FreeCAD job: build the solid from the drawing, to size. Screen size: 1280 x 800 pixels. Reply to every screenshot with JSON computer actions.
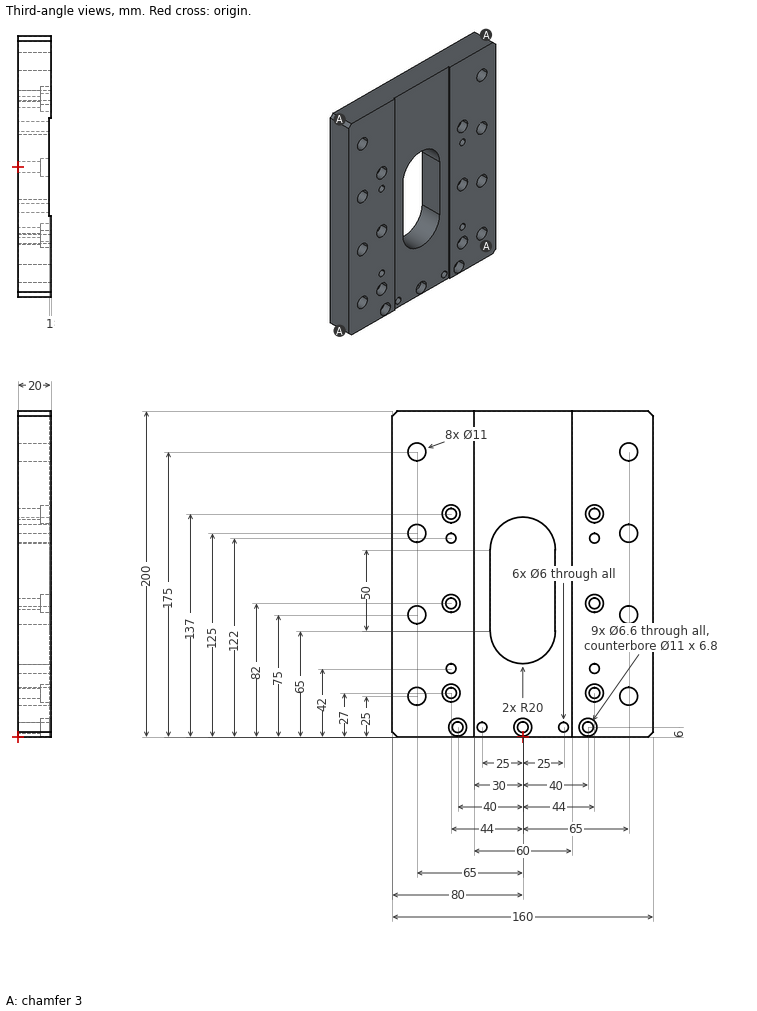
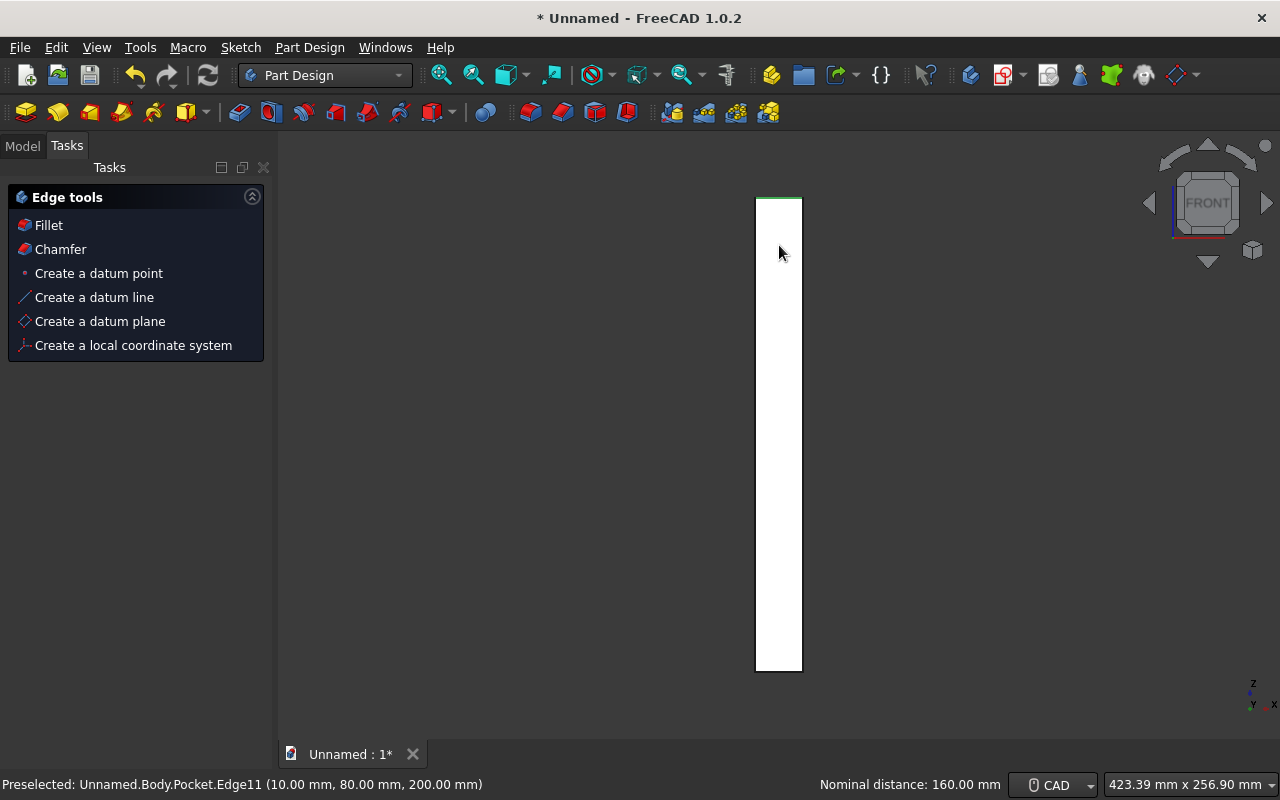
{"action": "left_click", "coordinate": [779, 671], "text": "ctrl"}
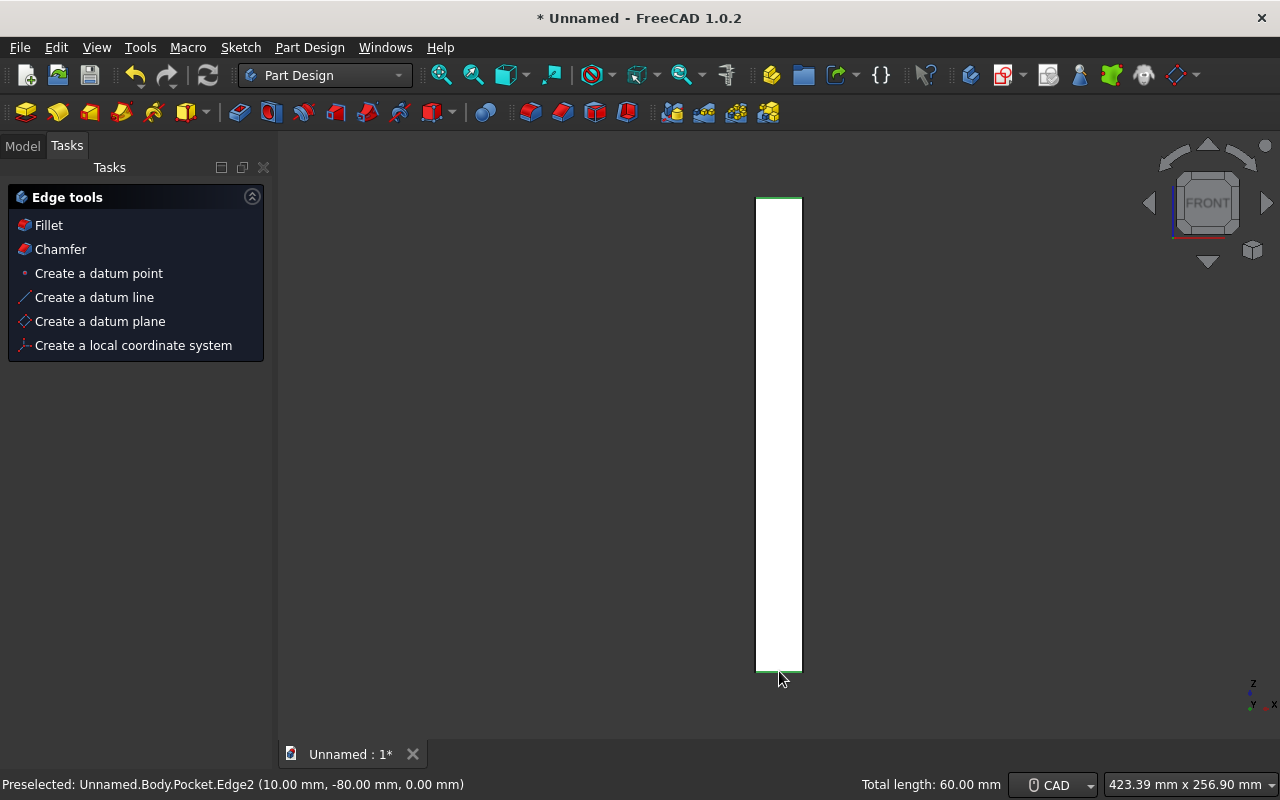
{"action": "key", "text": "3"}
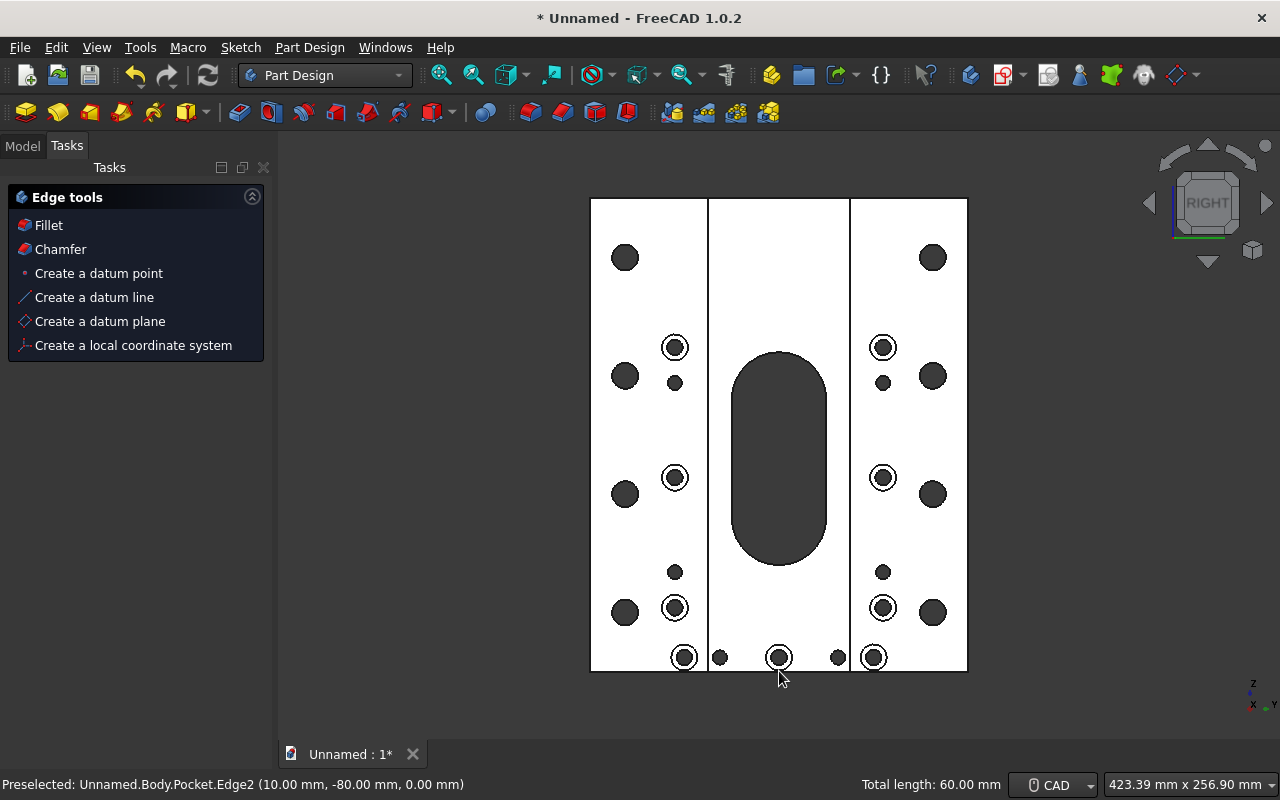
{"action": "key", "text": "5"}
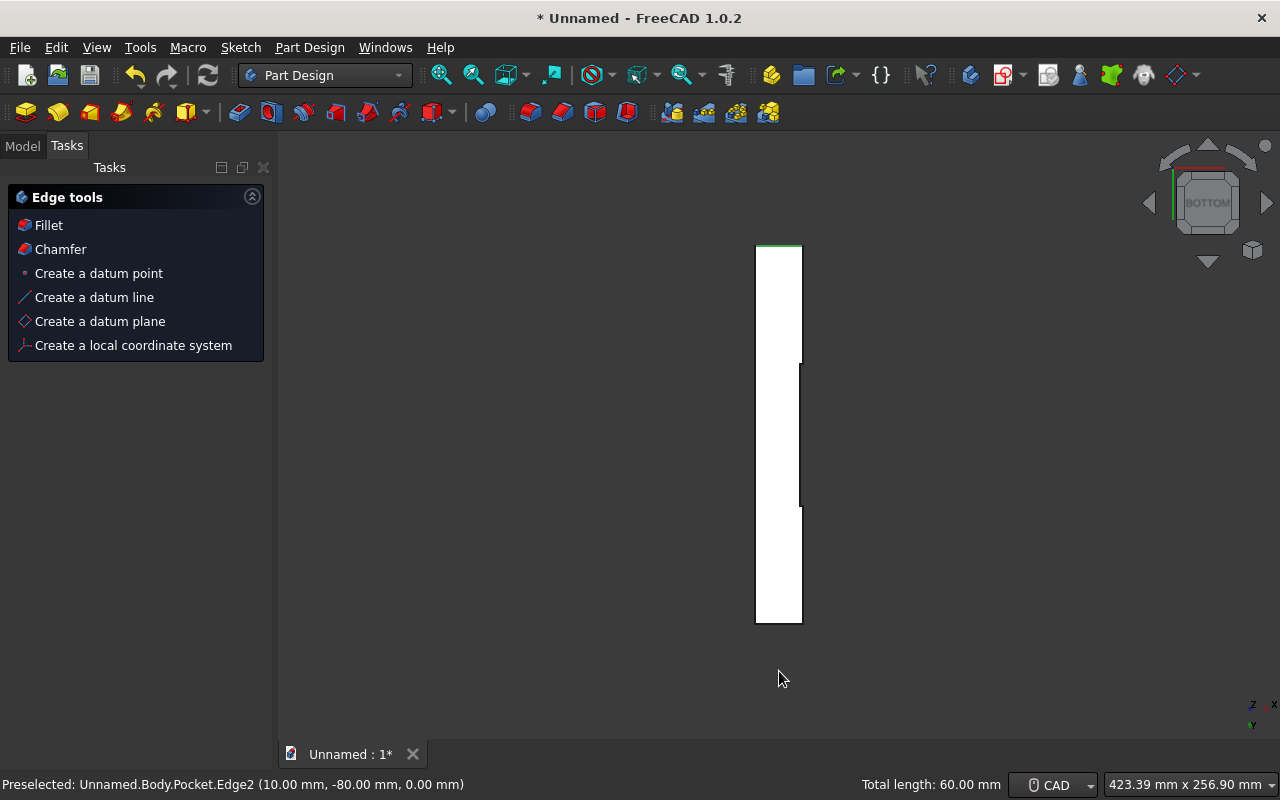
{"action": "left_click", "coordinate": [779, 623], "text": "ctrl"}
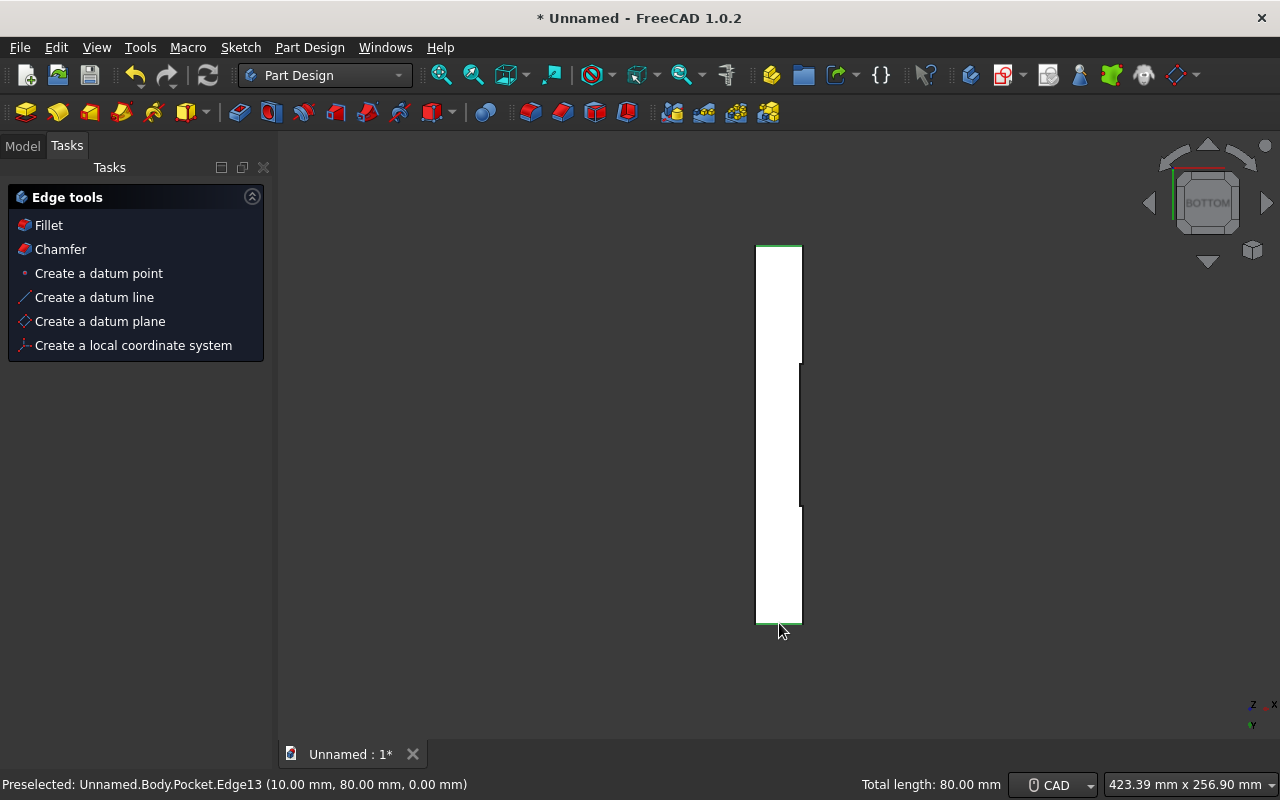
{"action": "left_click", "coordinate": [564, 112]}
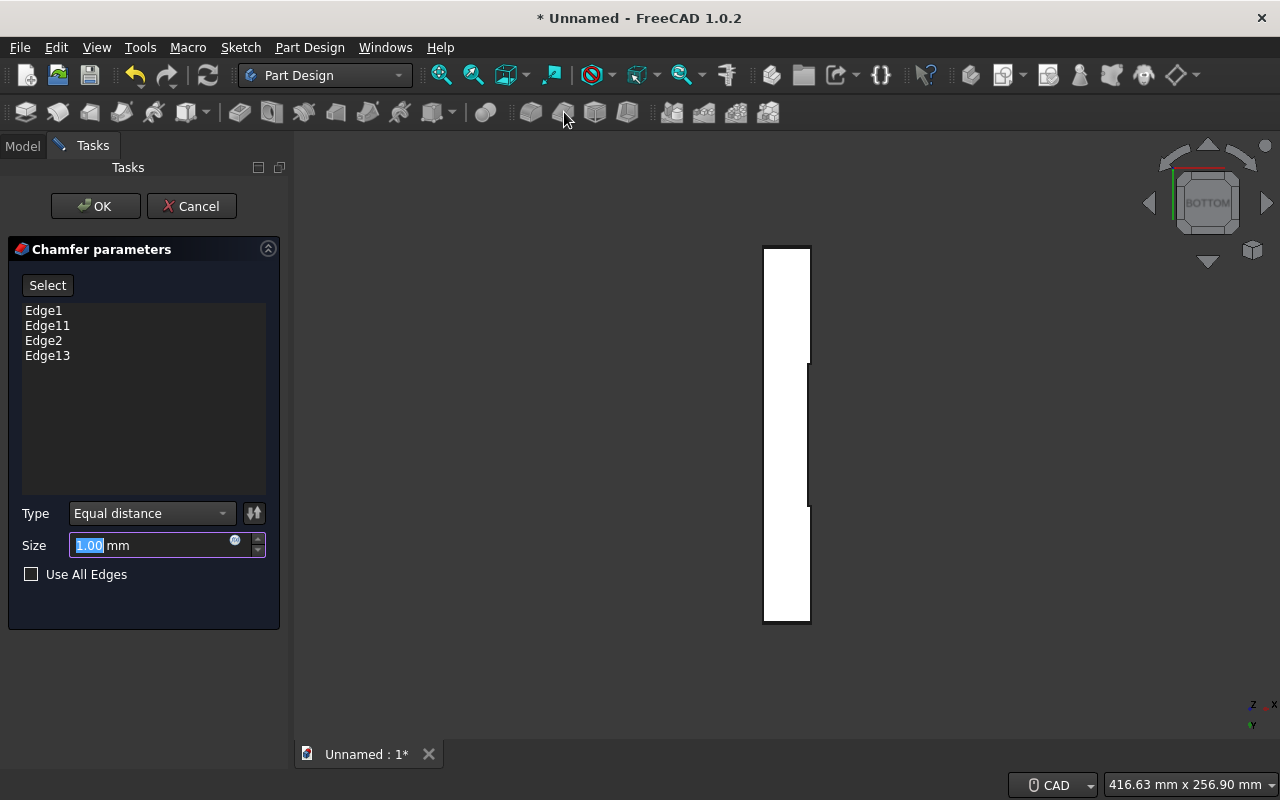
{"action": "type", "text": "3"}
{"action": "key", "text": "Tab"}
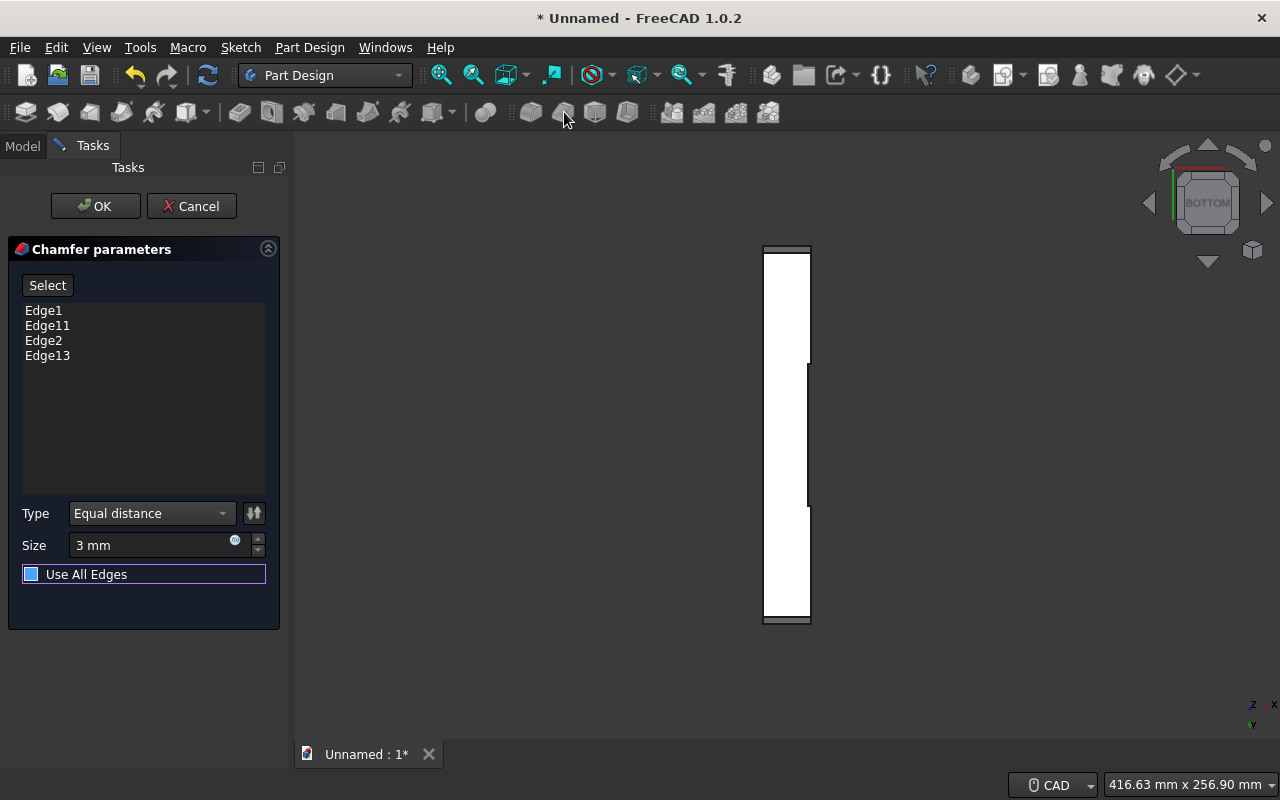
{"action": "left_click", "coordinate": [96, 206]}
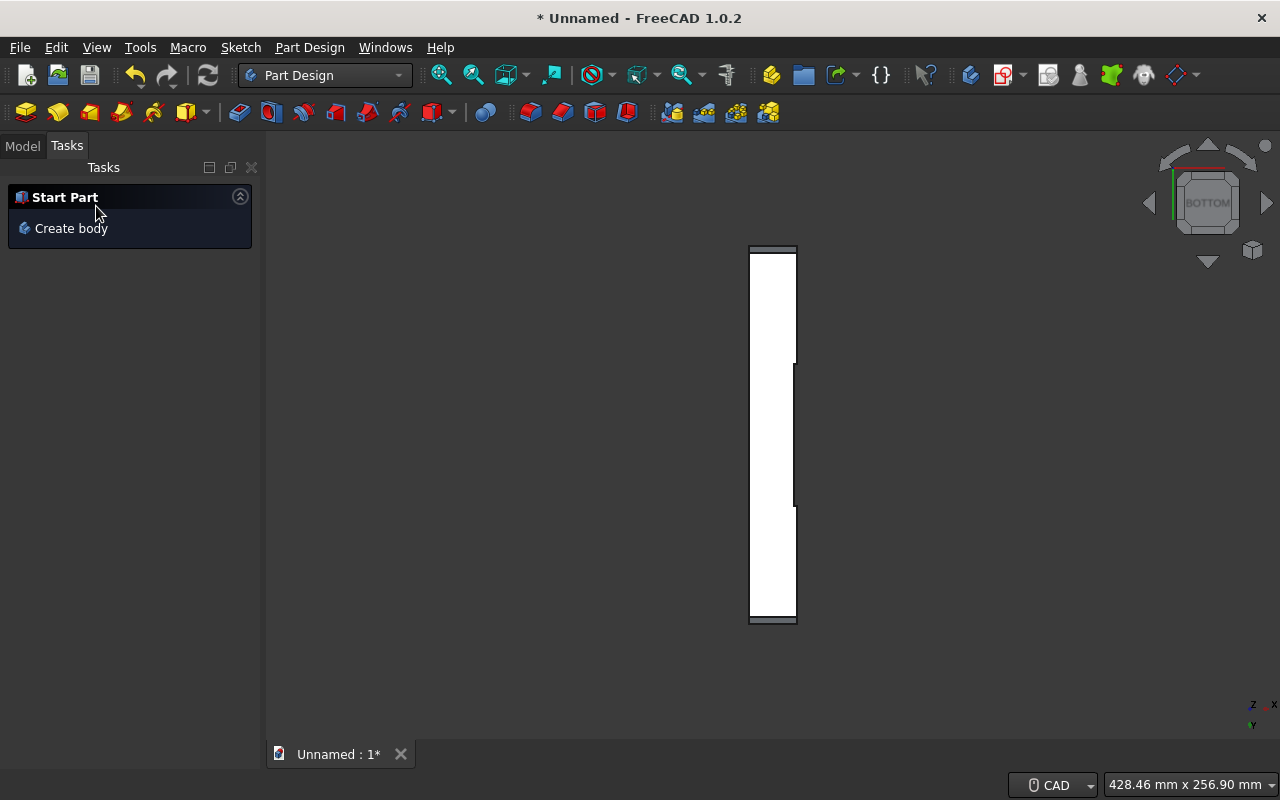
{"action": "key", "text": "0"}